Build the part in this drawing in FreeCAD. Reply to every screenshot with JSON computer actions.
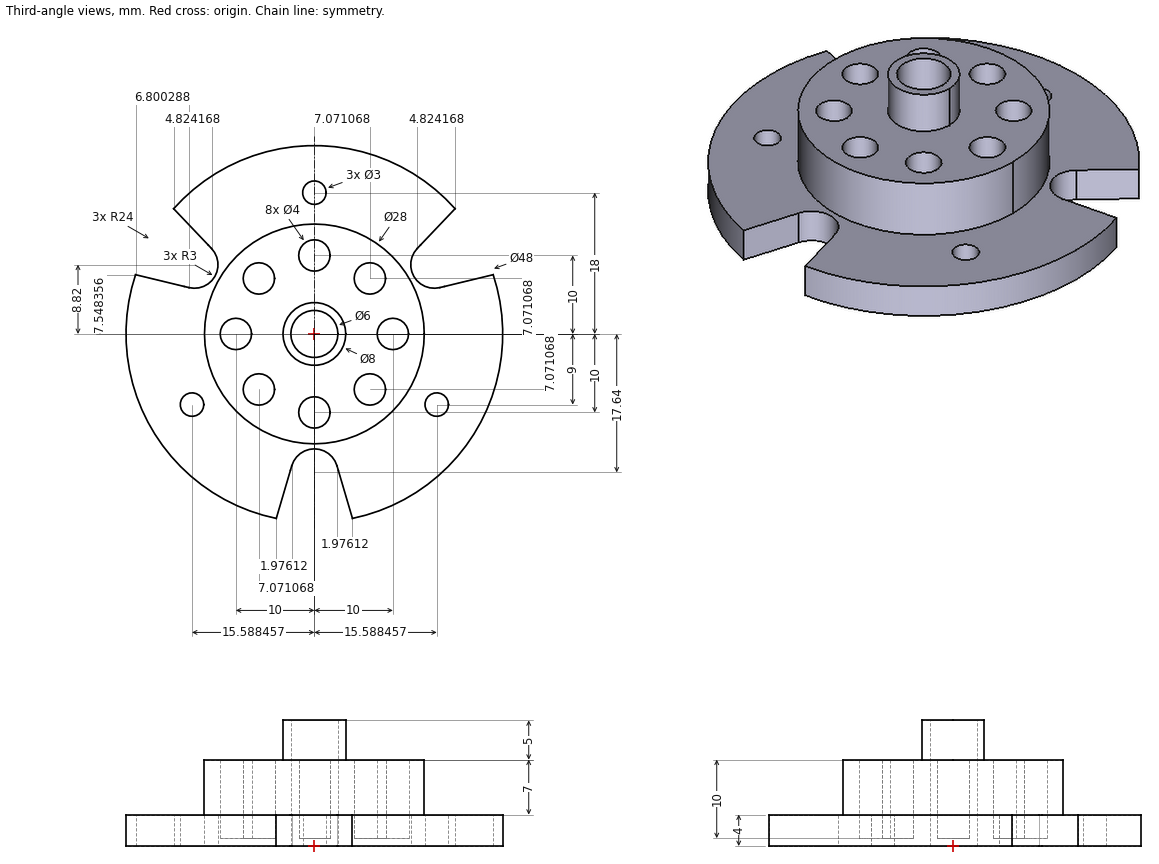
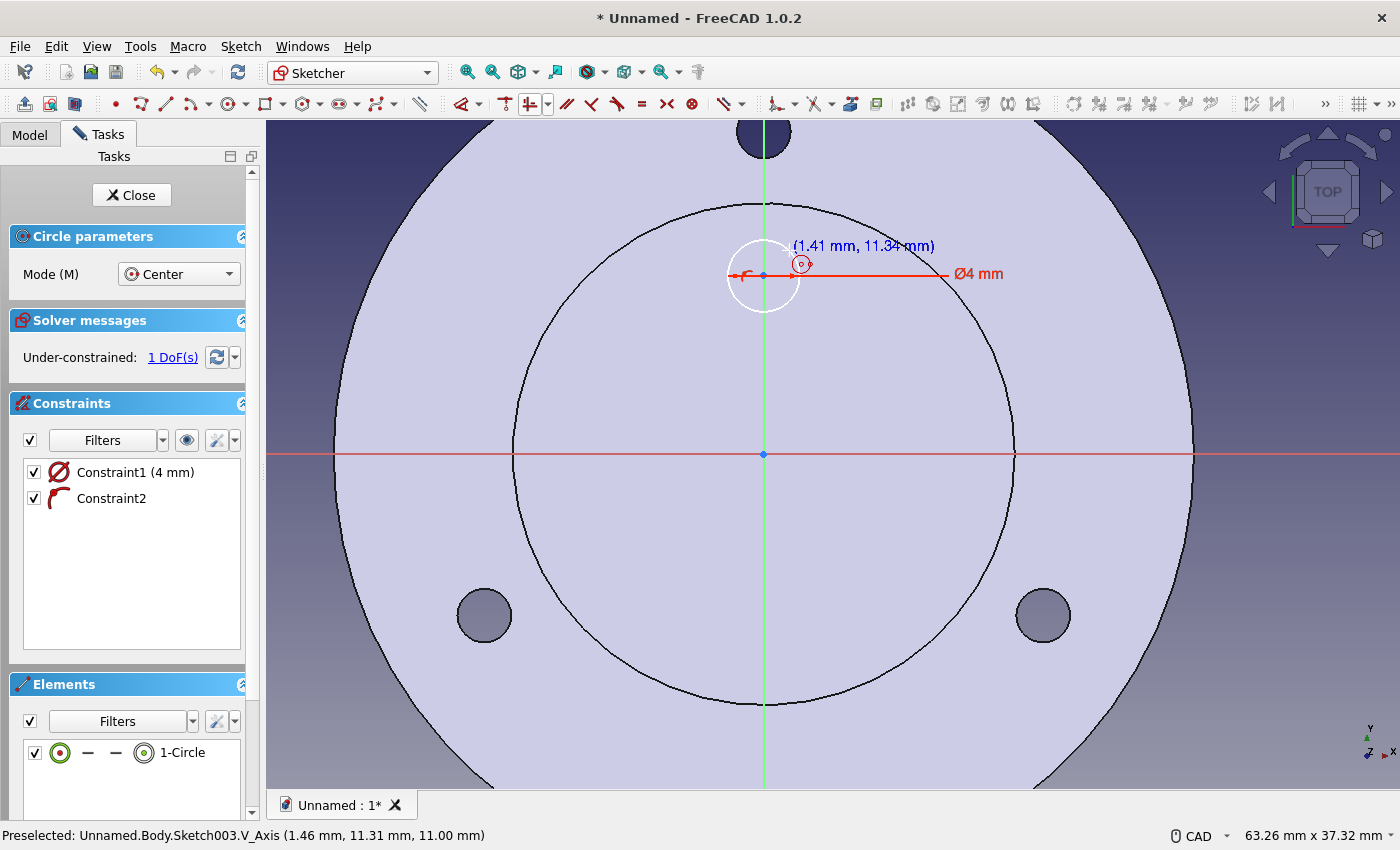
{"action": "left_click", "coordinate": [891, 327]}
{"action": "mouse_move", "coordinate": [916, 302]}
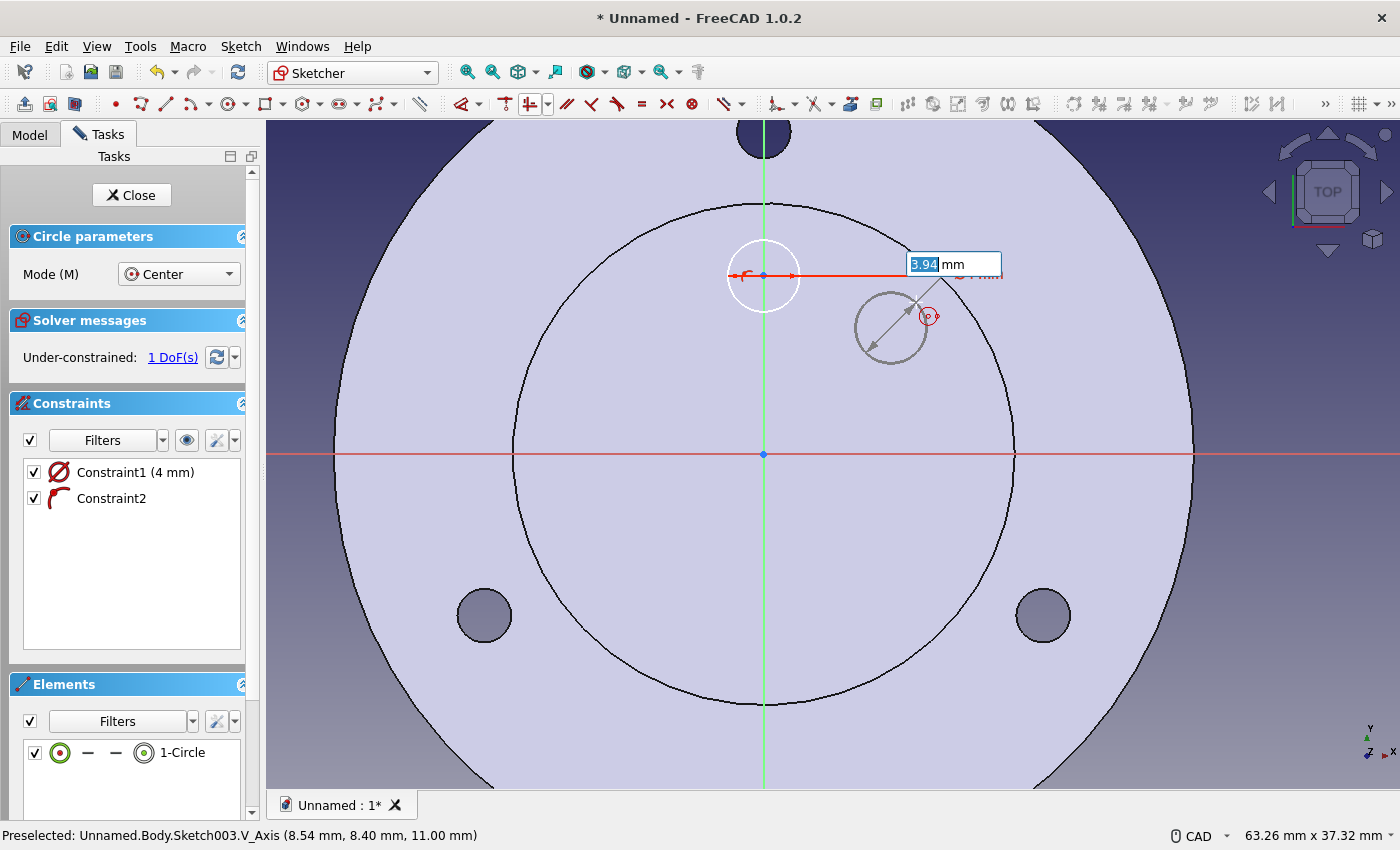
{"action": "type", "text": "4"}
{"action": "key", "text": "Return"}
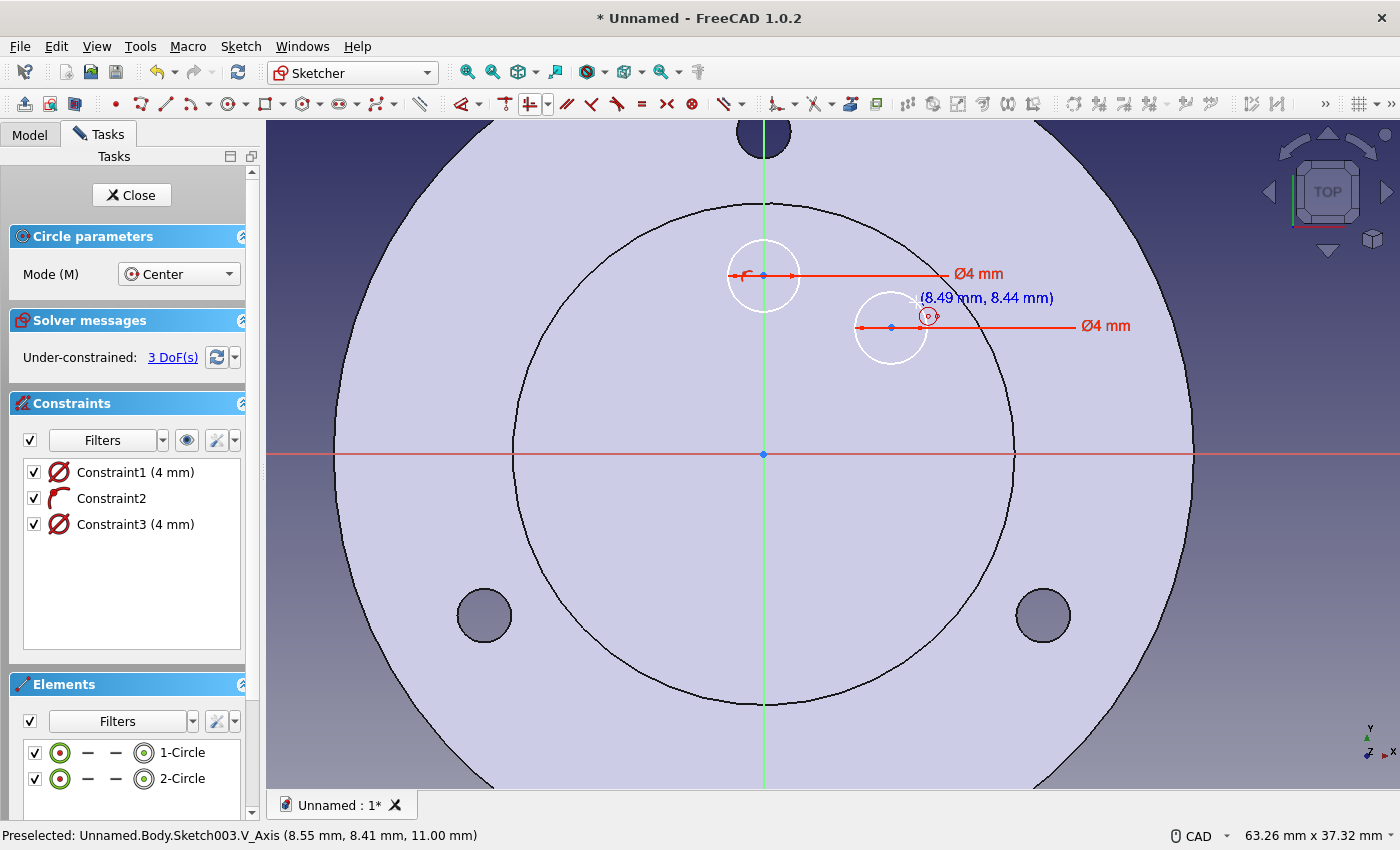
{"action": "left_click", "coordinate": [943, 454]}
{"action": "mouse_move", "coordinate": [968, 429]}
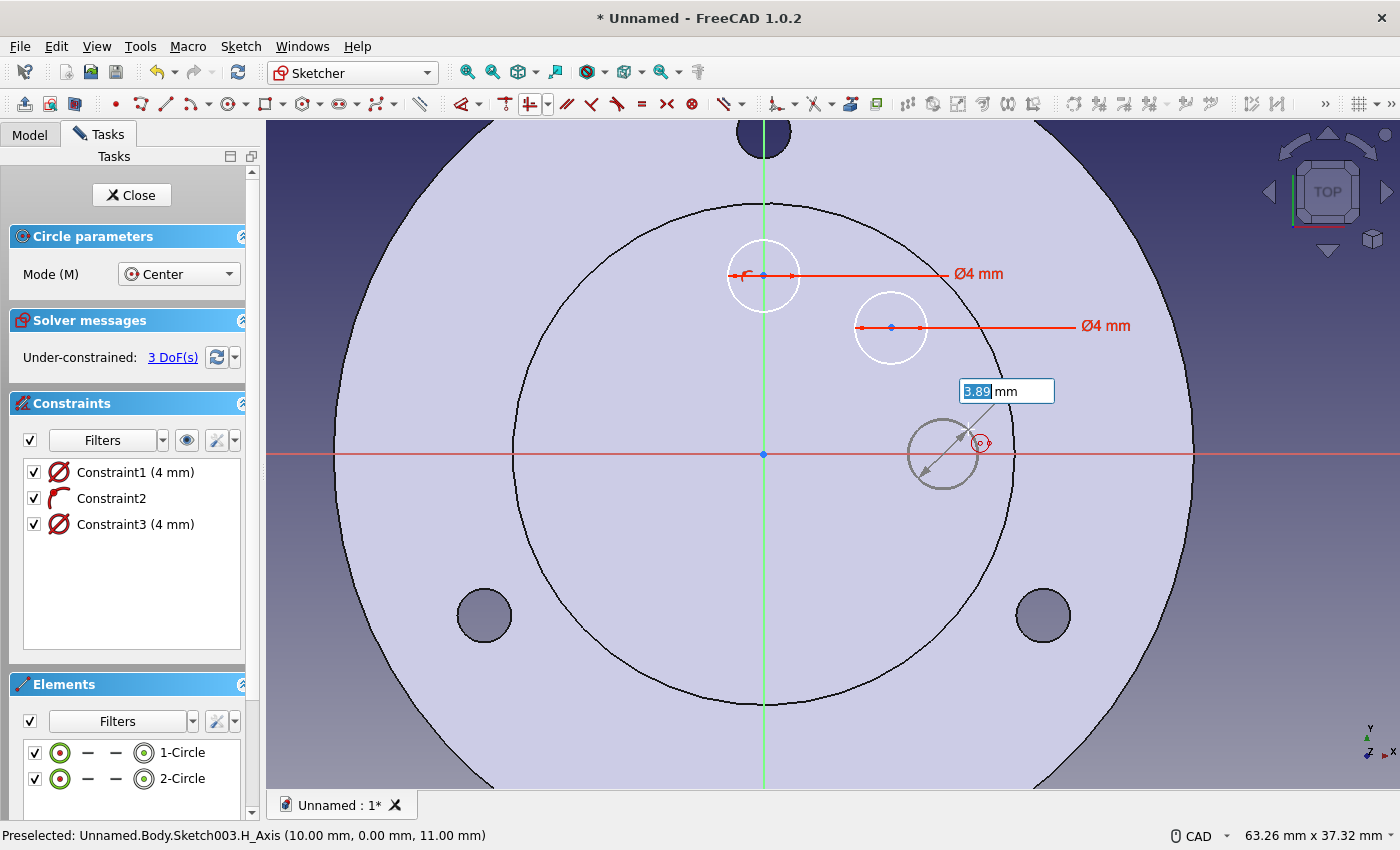
{"action": "type", "text": "4"}
{"action": "key", "text": "Return"}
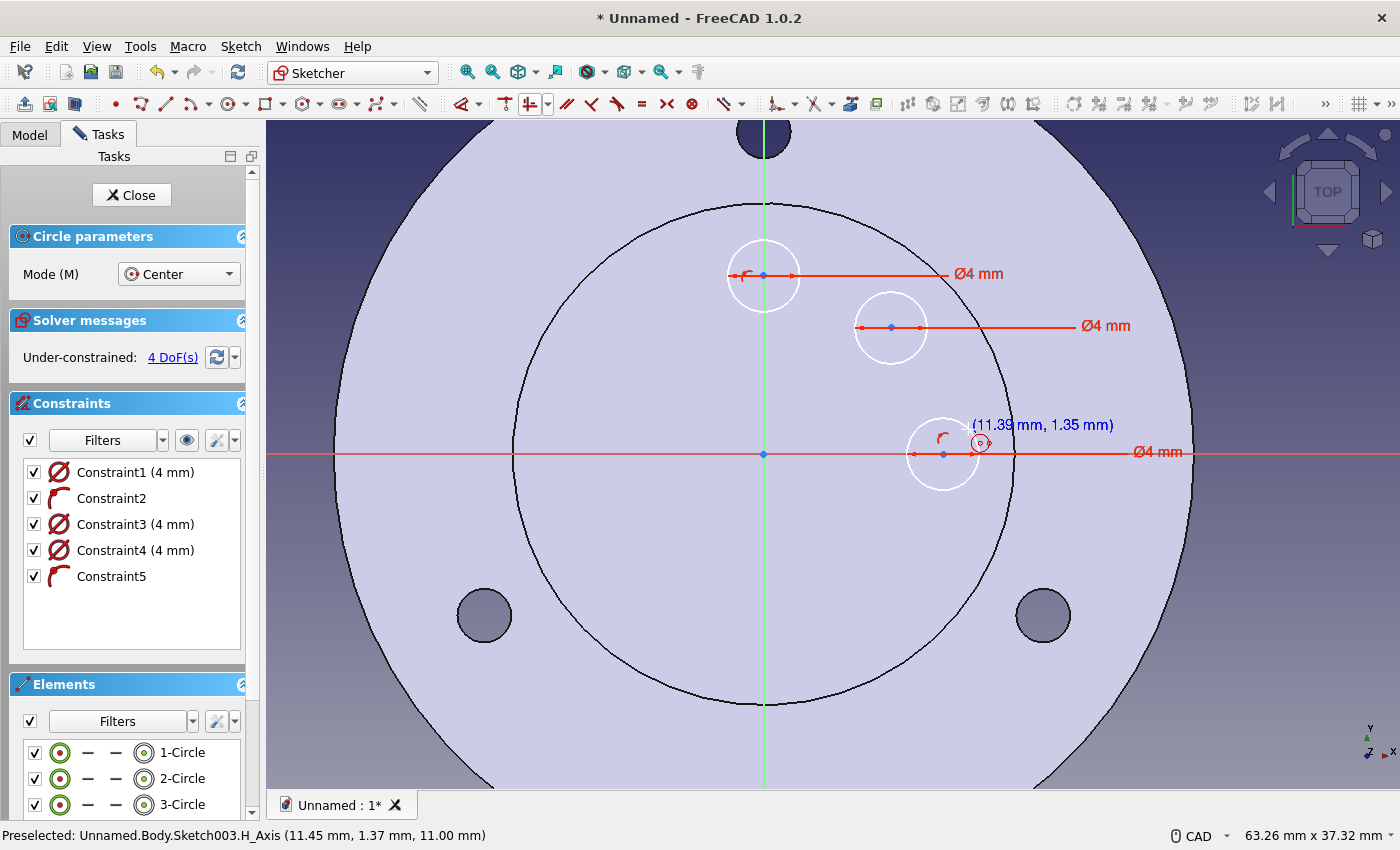
{"action": "left_click", "coordinate": [891, 581]}
{"action": "mouse_move", "coordinate": [916, 556]}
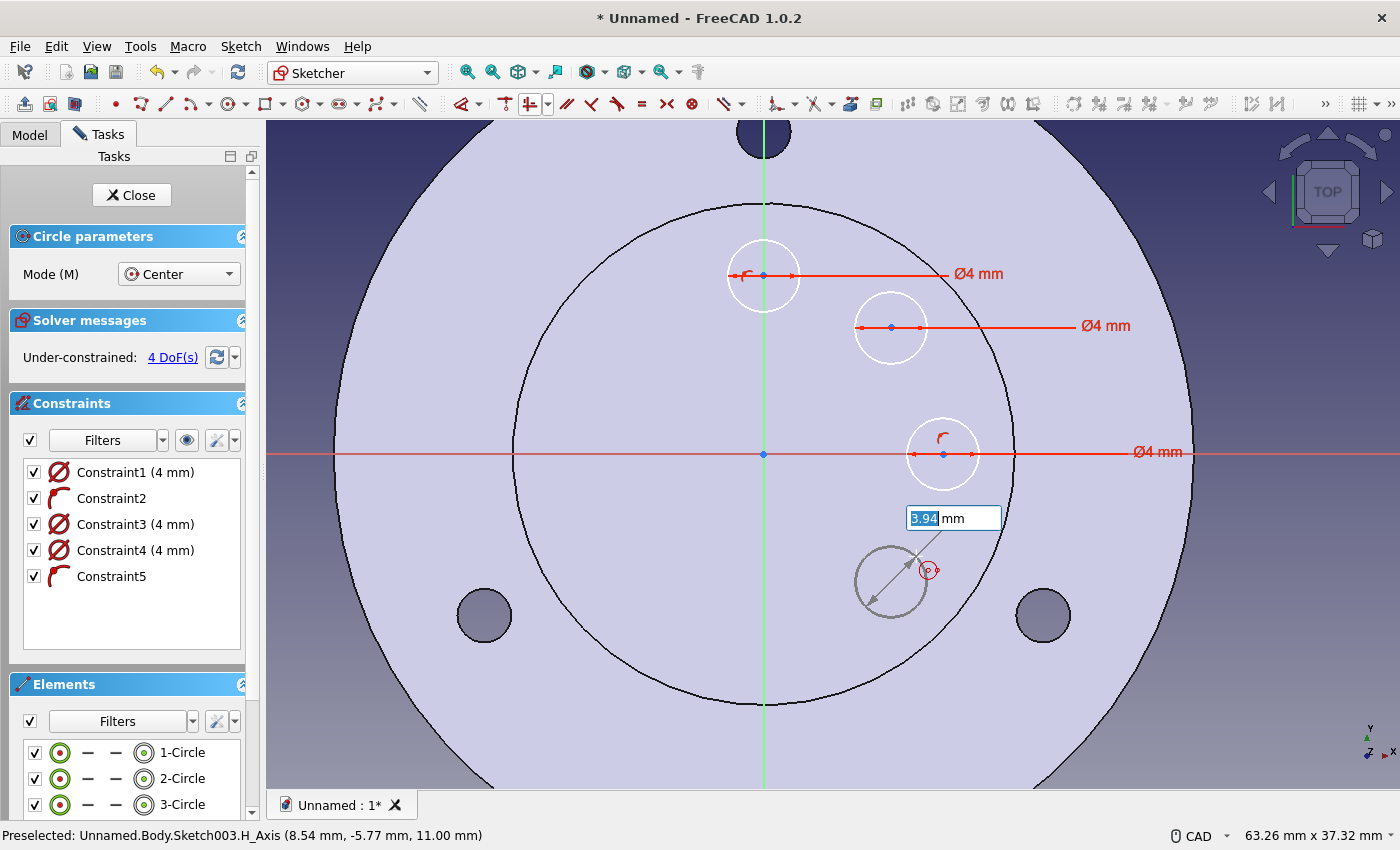
{"action": "type", "text": "4"}
{"action": "key", "text": "Return"}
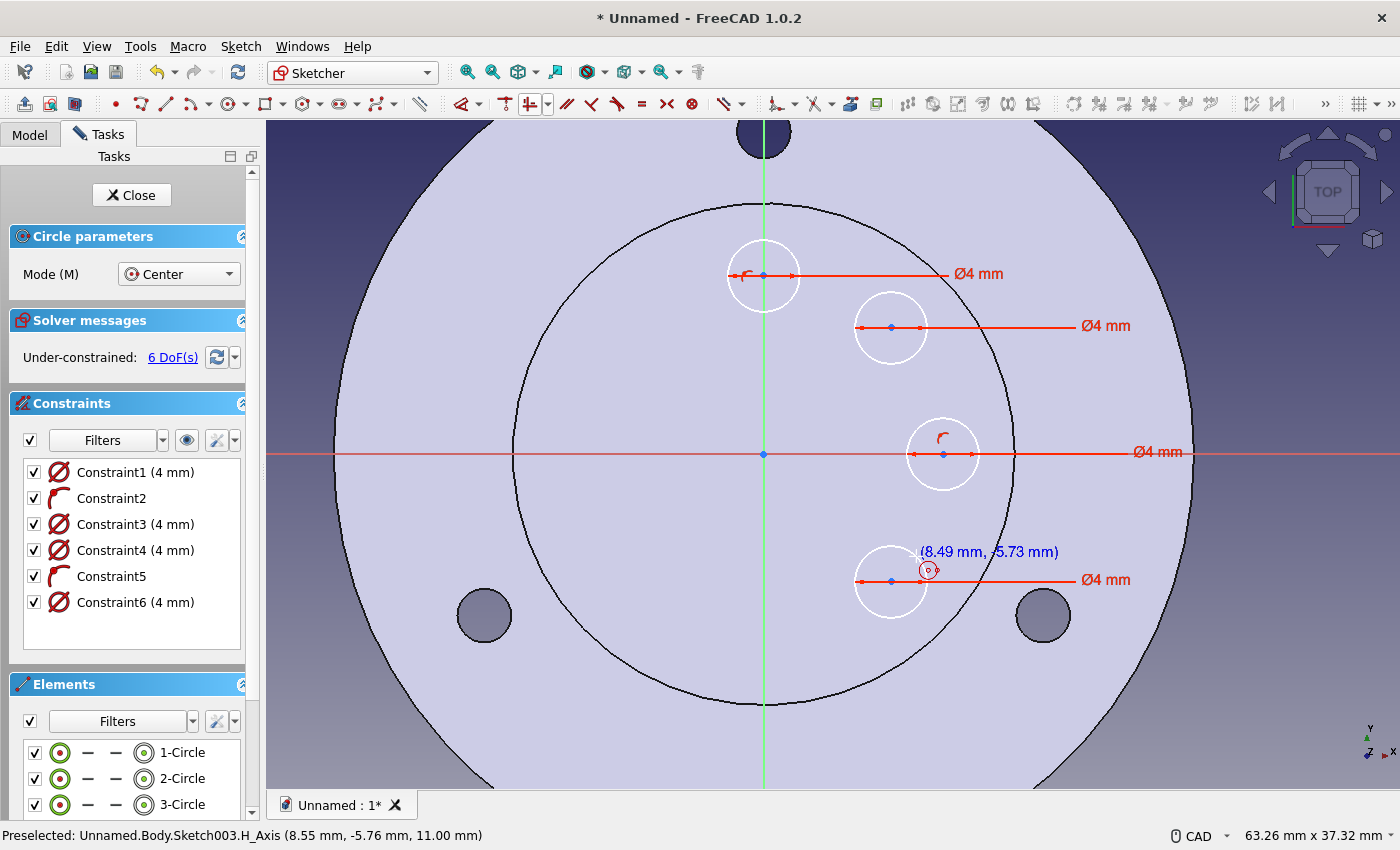
{"action": "left_click", "coordinate": [764, 634]}
{"action": "mouse_move", "coordinate": [789, 608]}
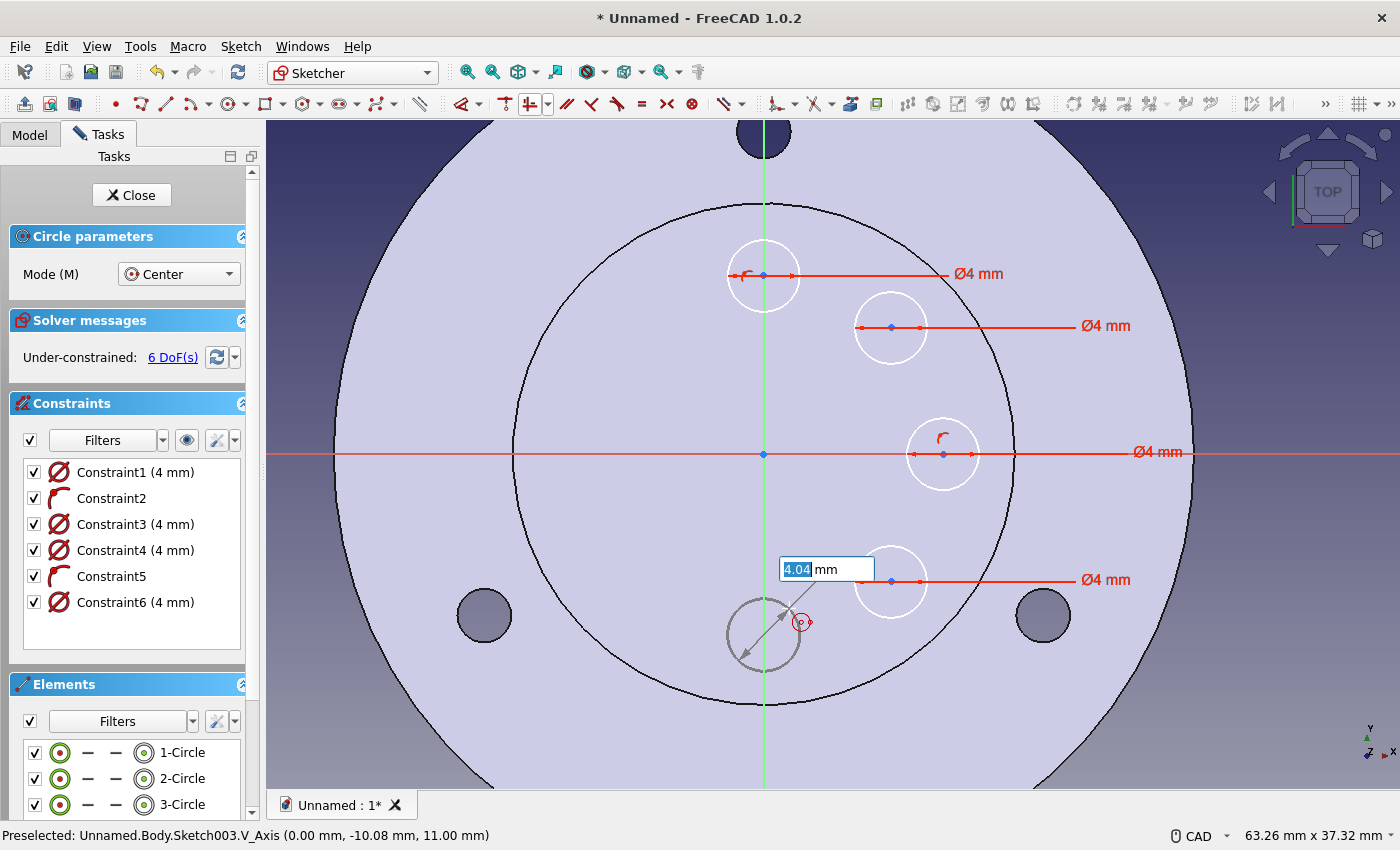
{"action": "type", "text": "4"}
{"action": "key", "text": "Return"}